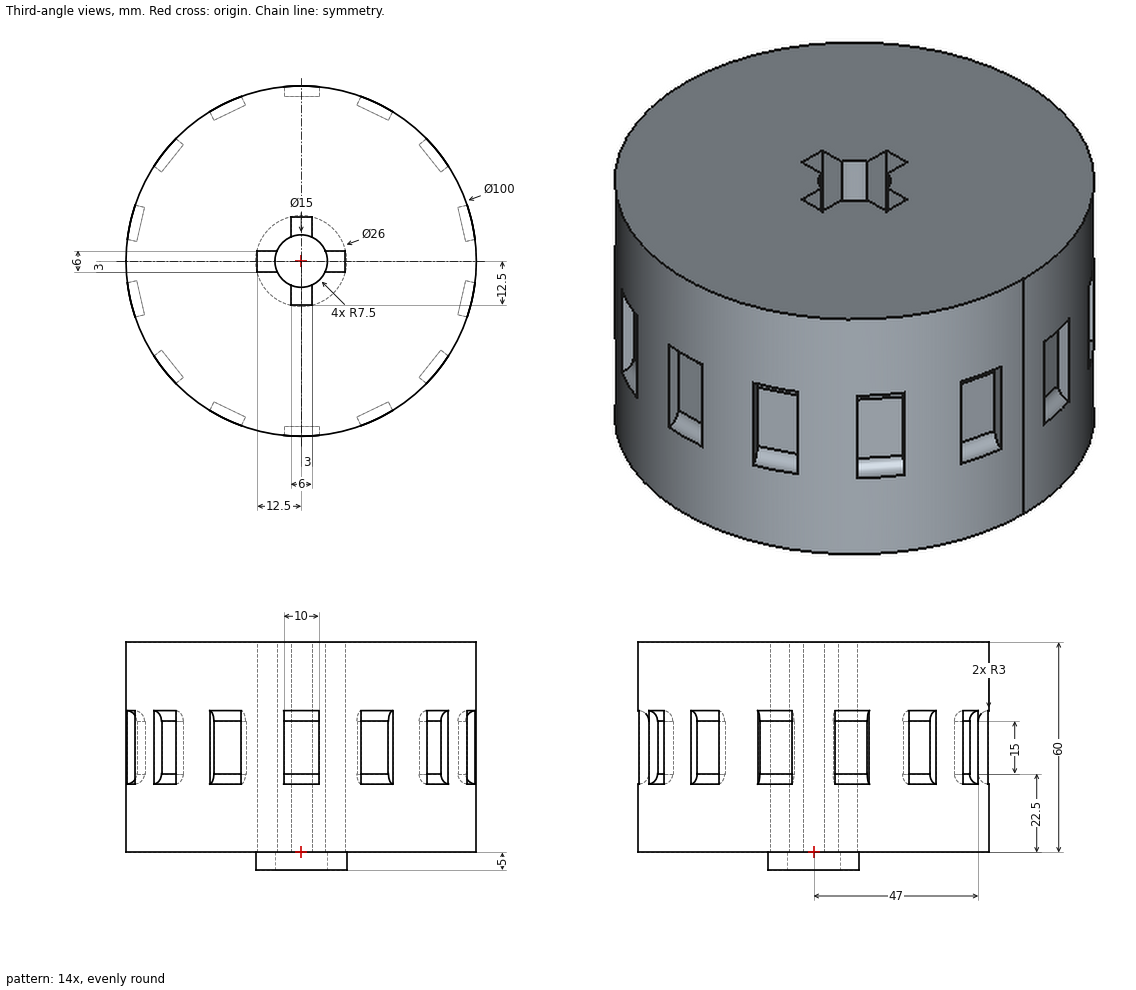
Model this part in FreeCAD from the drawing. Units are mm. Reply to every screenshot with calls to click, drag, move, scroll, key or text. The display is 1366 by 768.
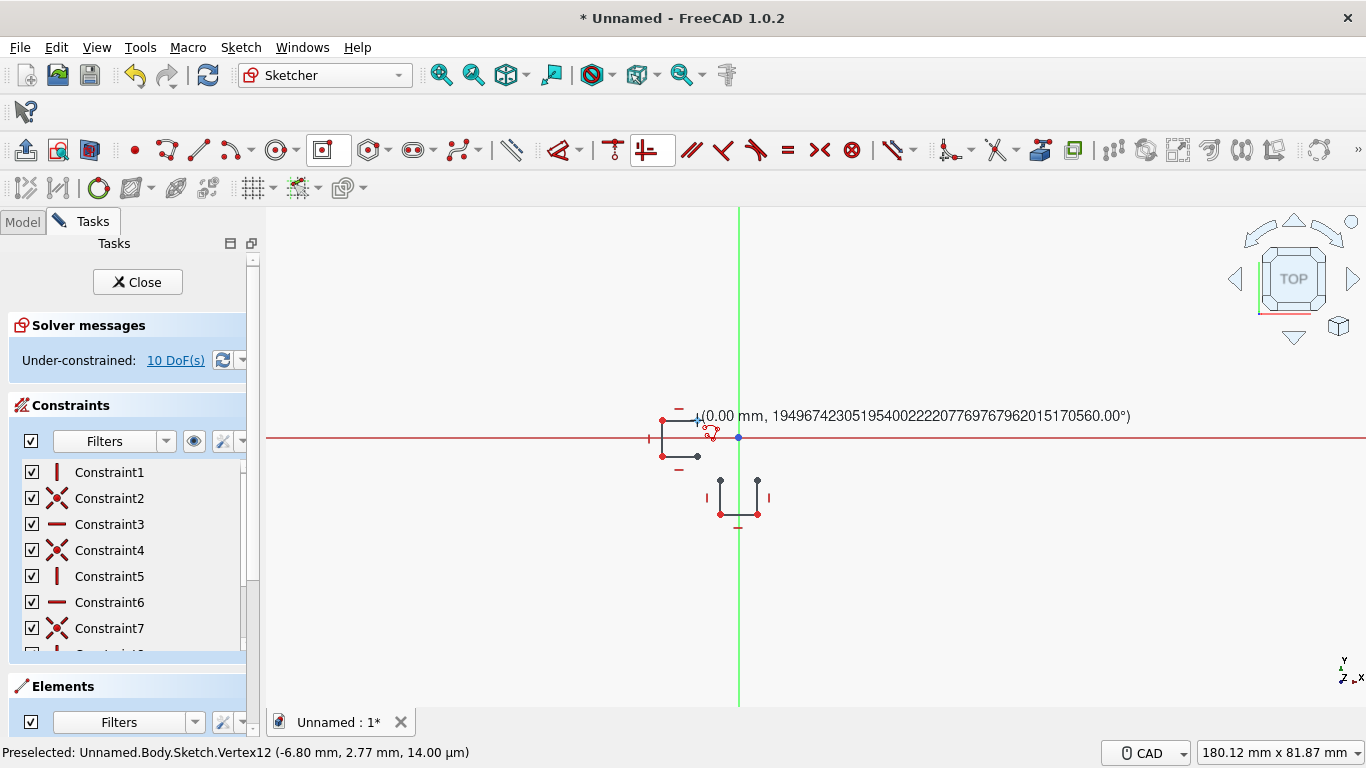
click(720, 396)
click(720, 362)
click(757, 362)
click(757, 396)
right_click(757, 396)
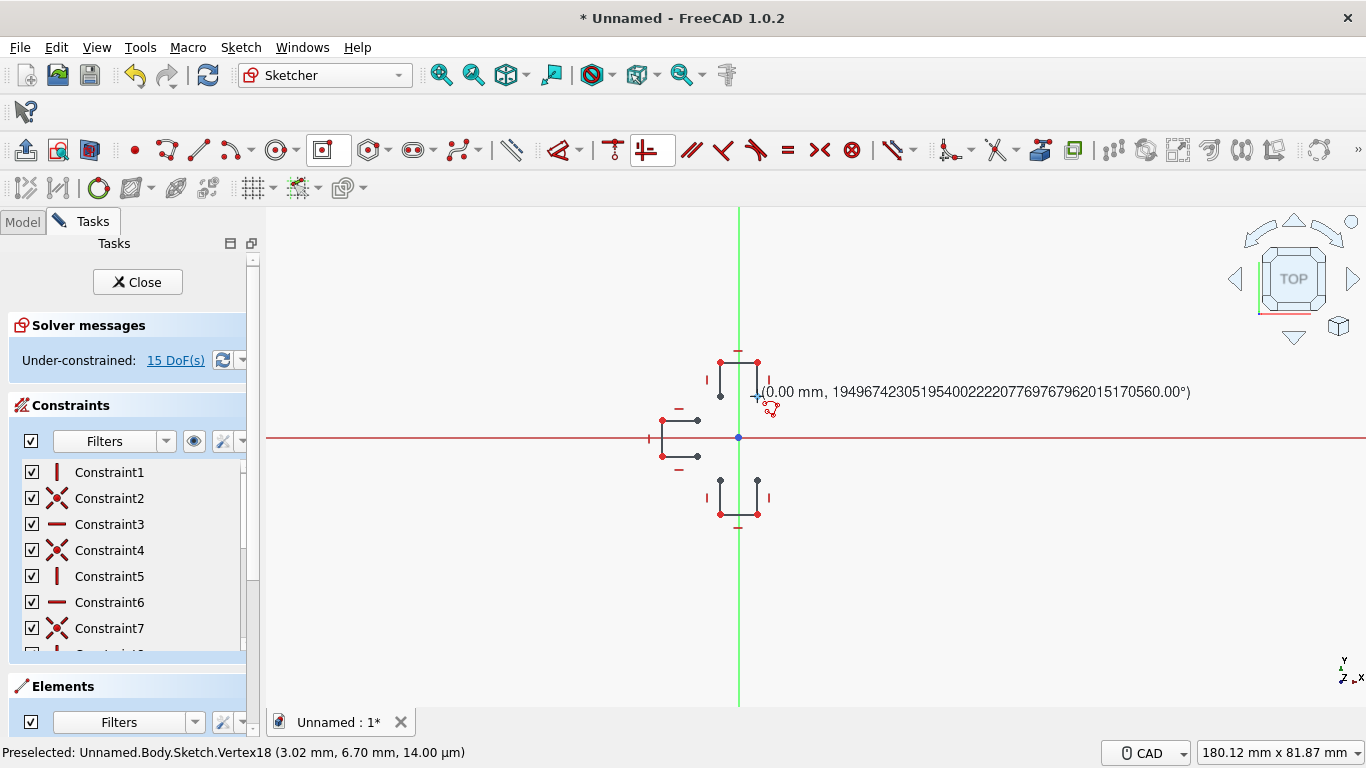
click(781, 420)
click(815, 420)
click(815, 456)
click(781, 456)
right_click(781, 456)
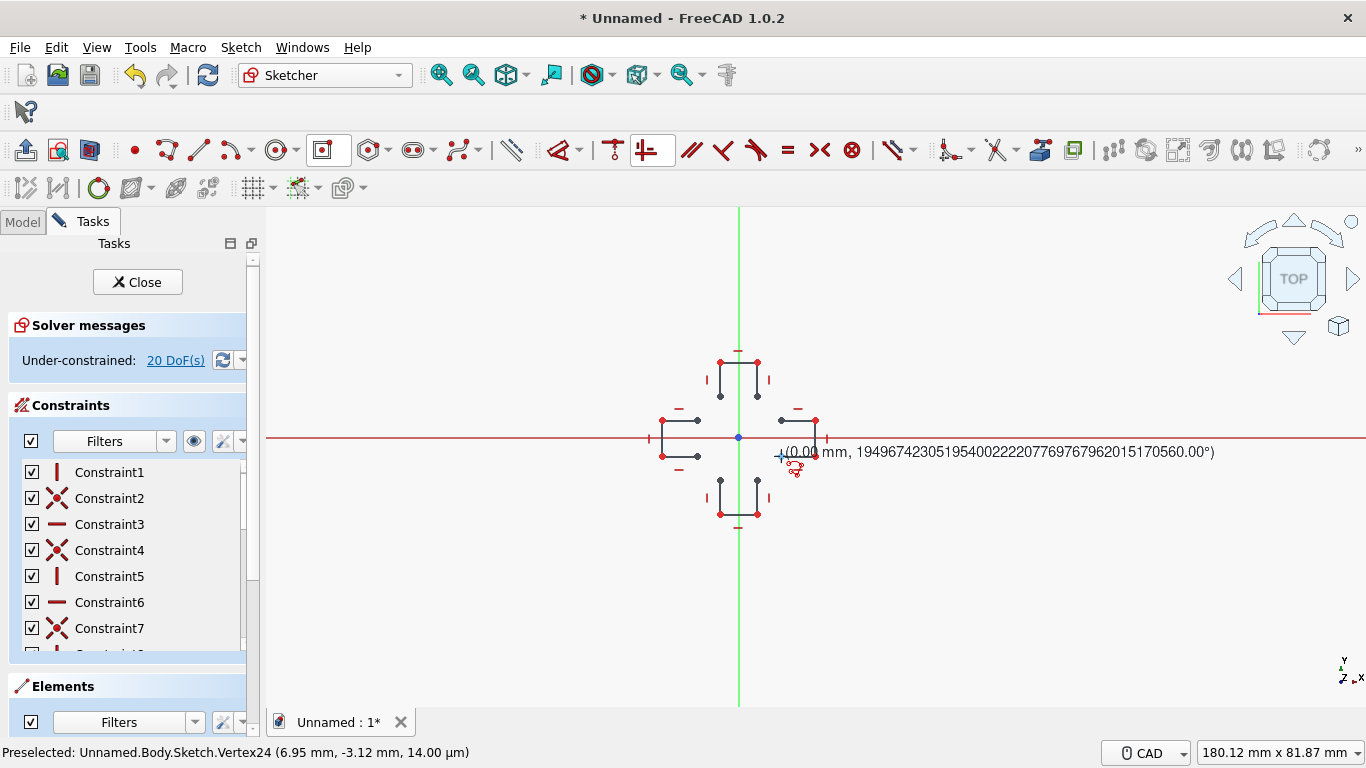
key(g)
key(3)
key(a)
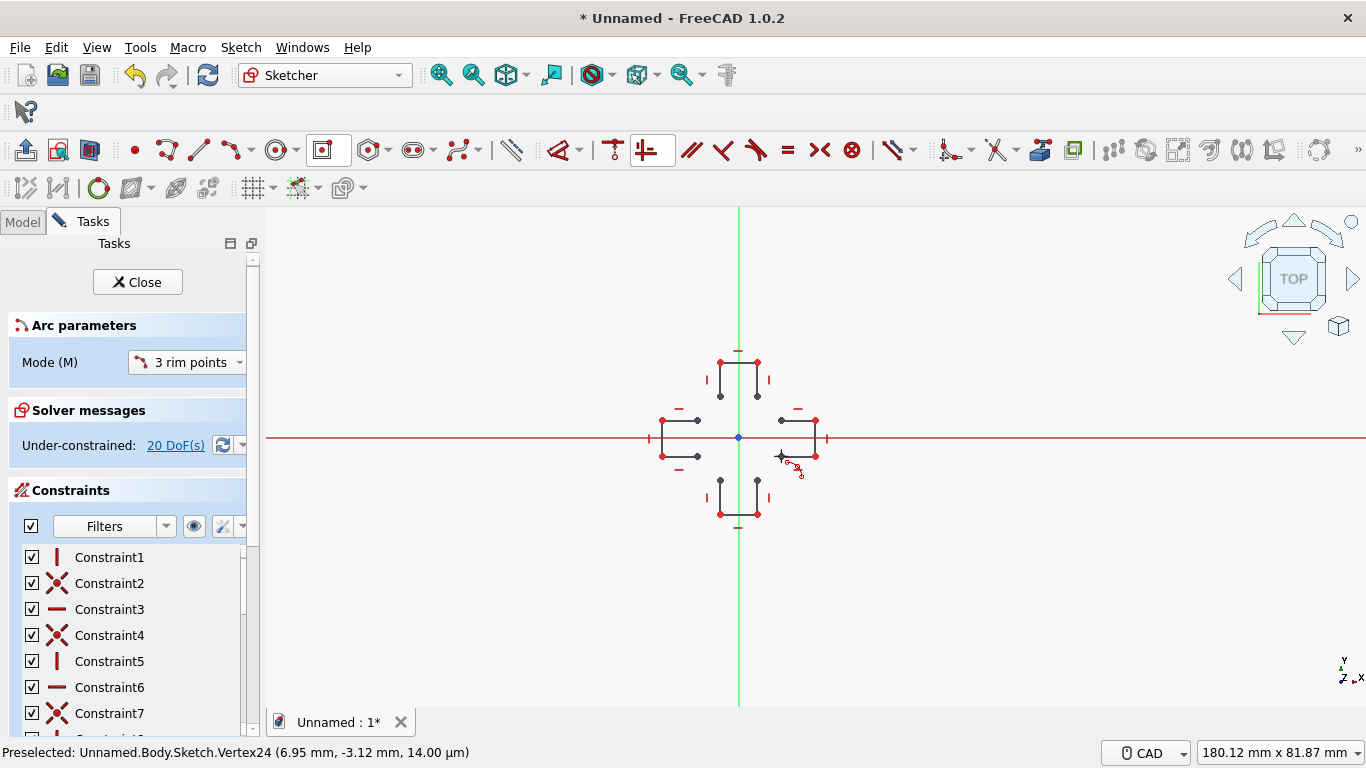
click(720, 481)
click(697, 457)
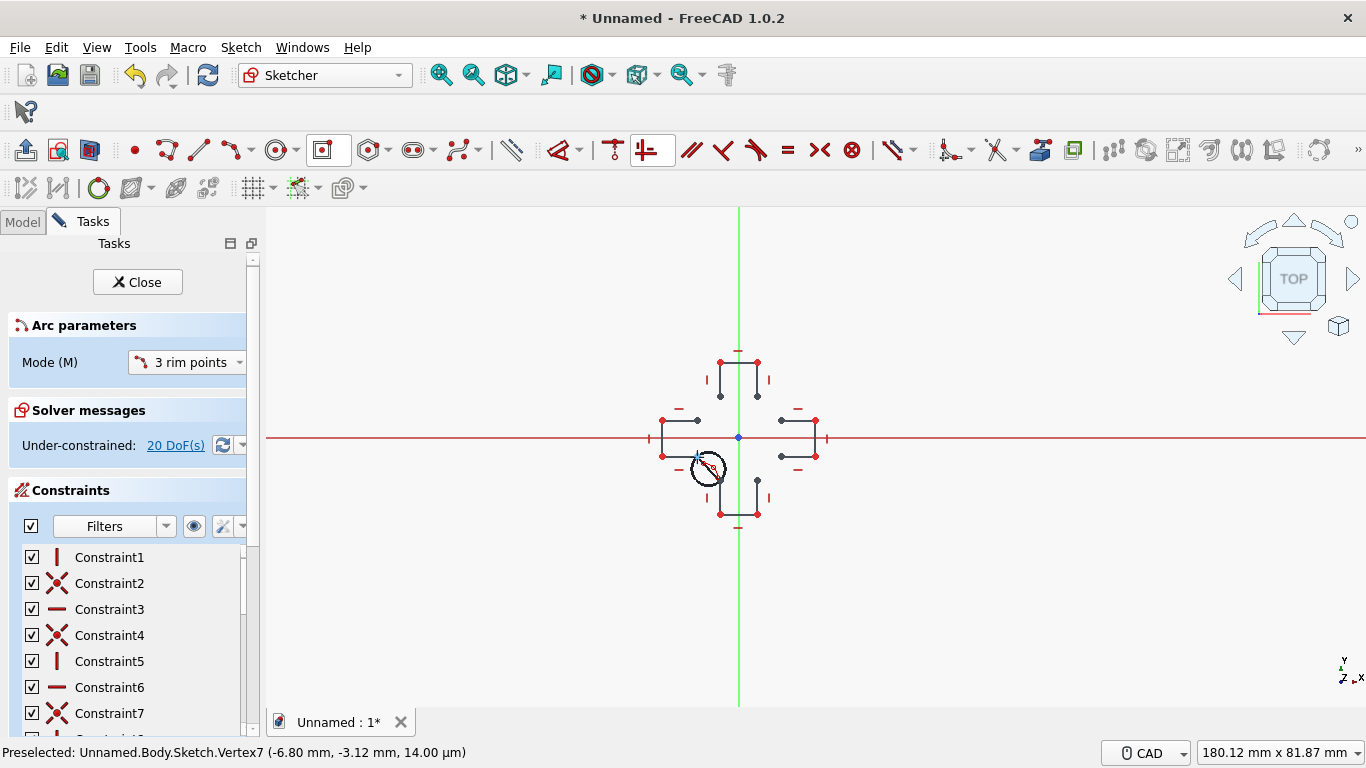
scroll(706, 470, up, 9)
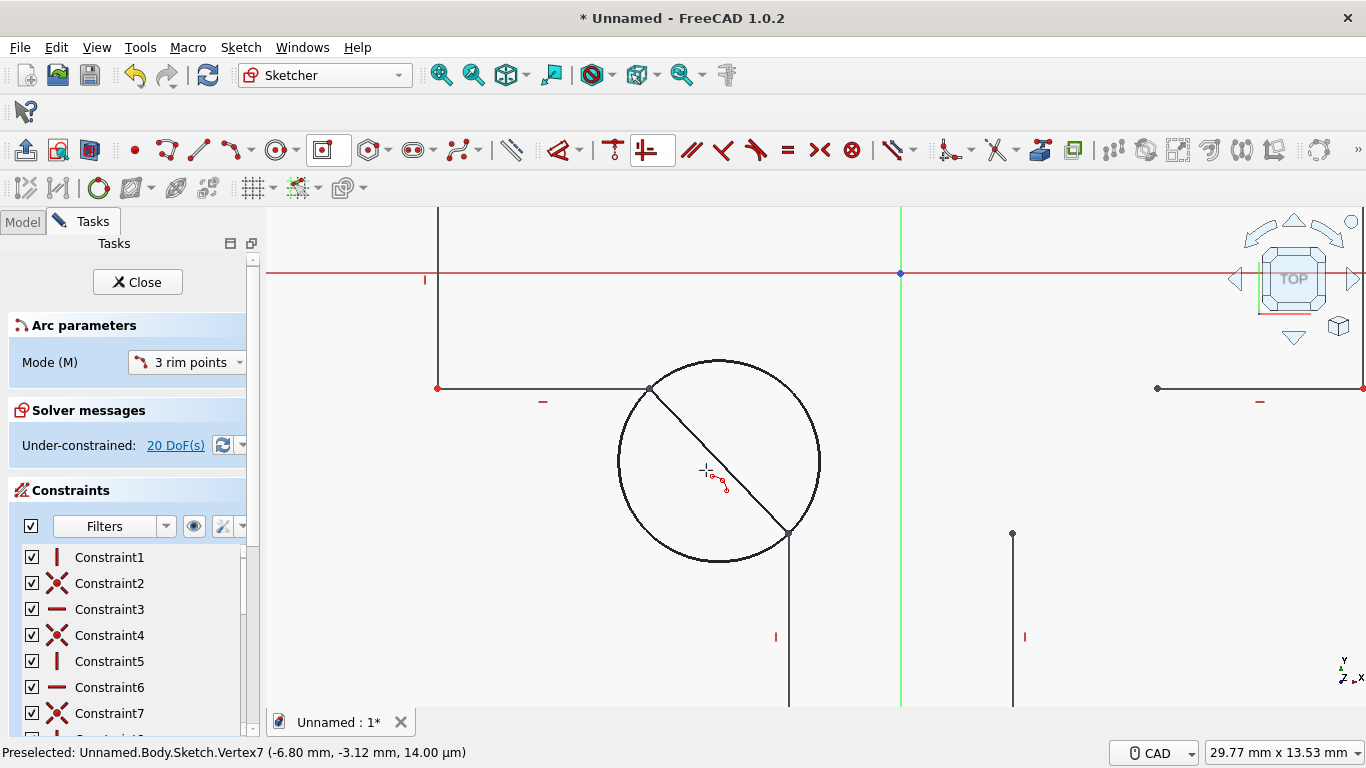
click(705, 469)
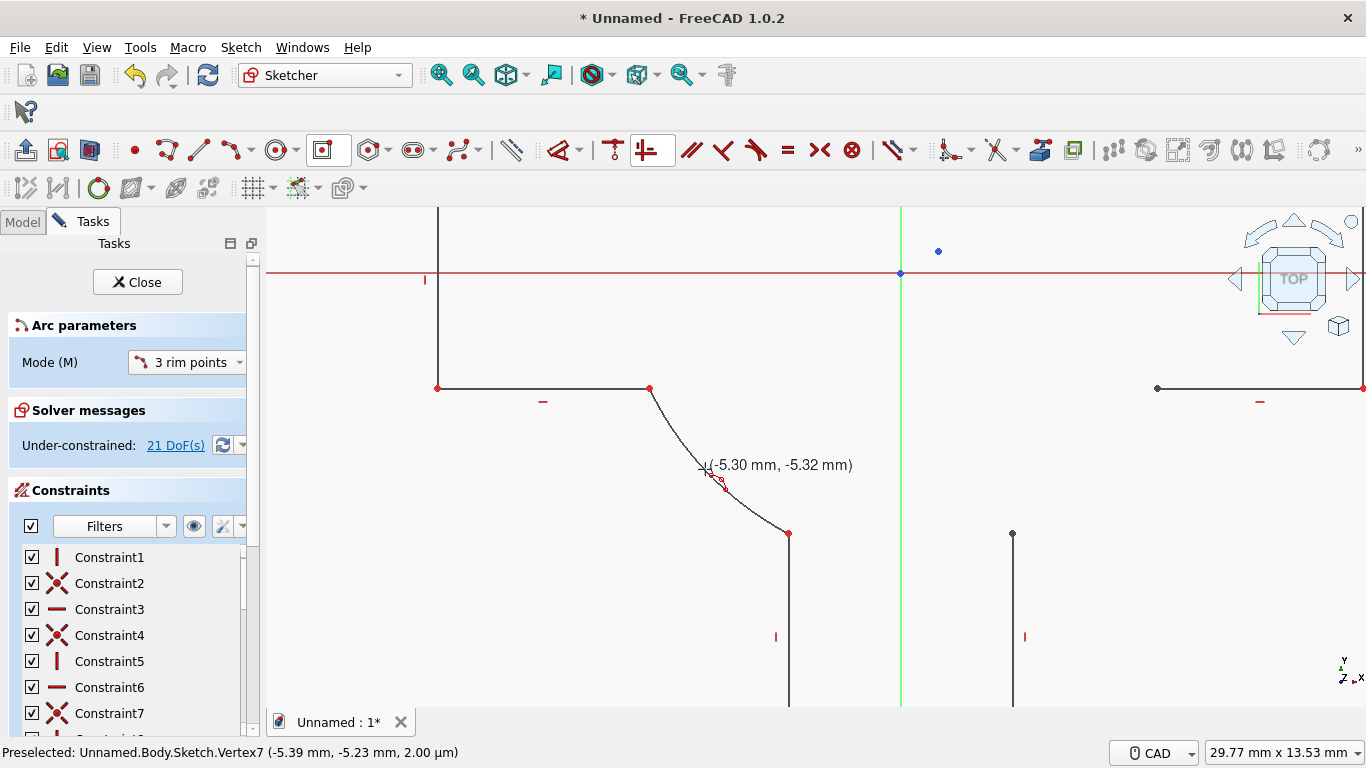
scroll(732, 475, down, 12)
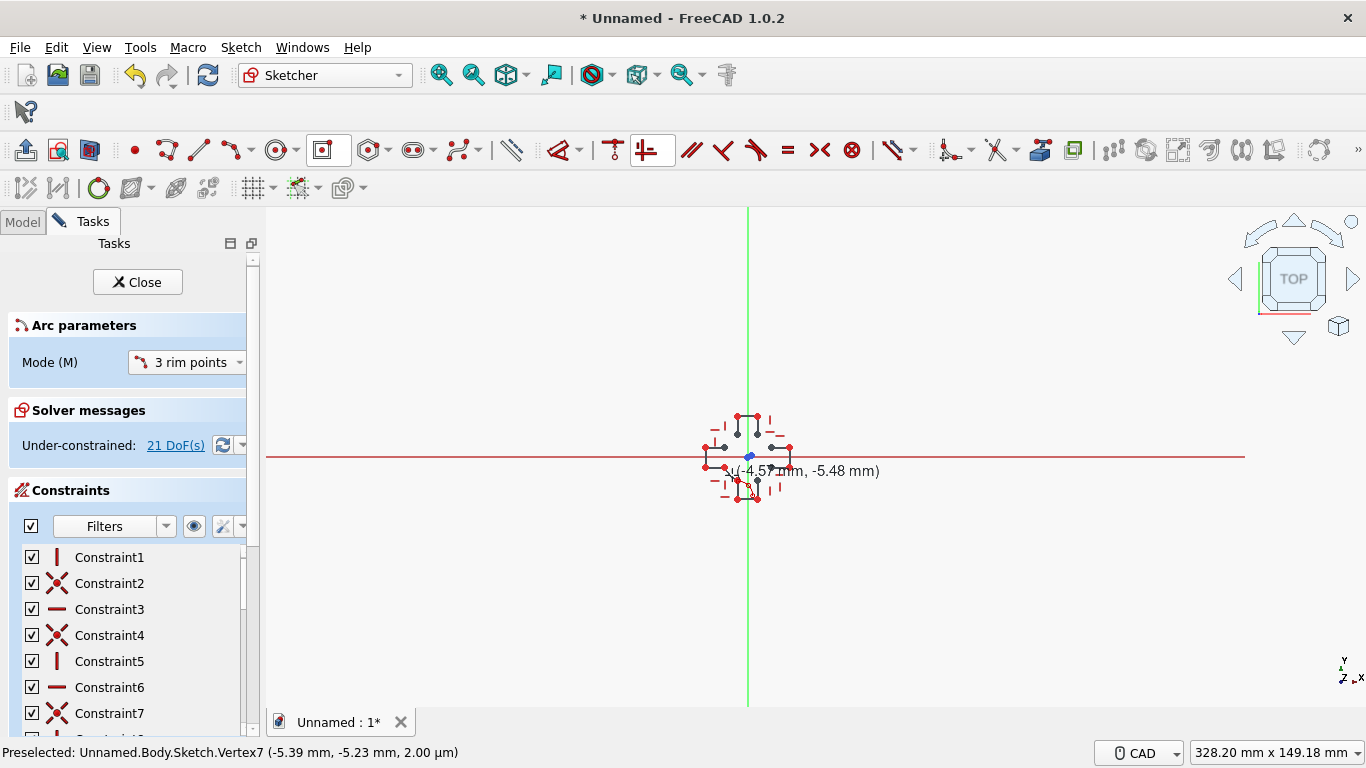
scroll(725, 447, up, 3)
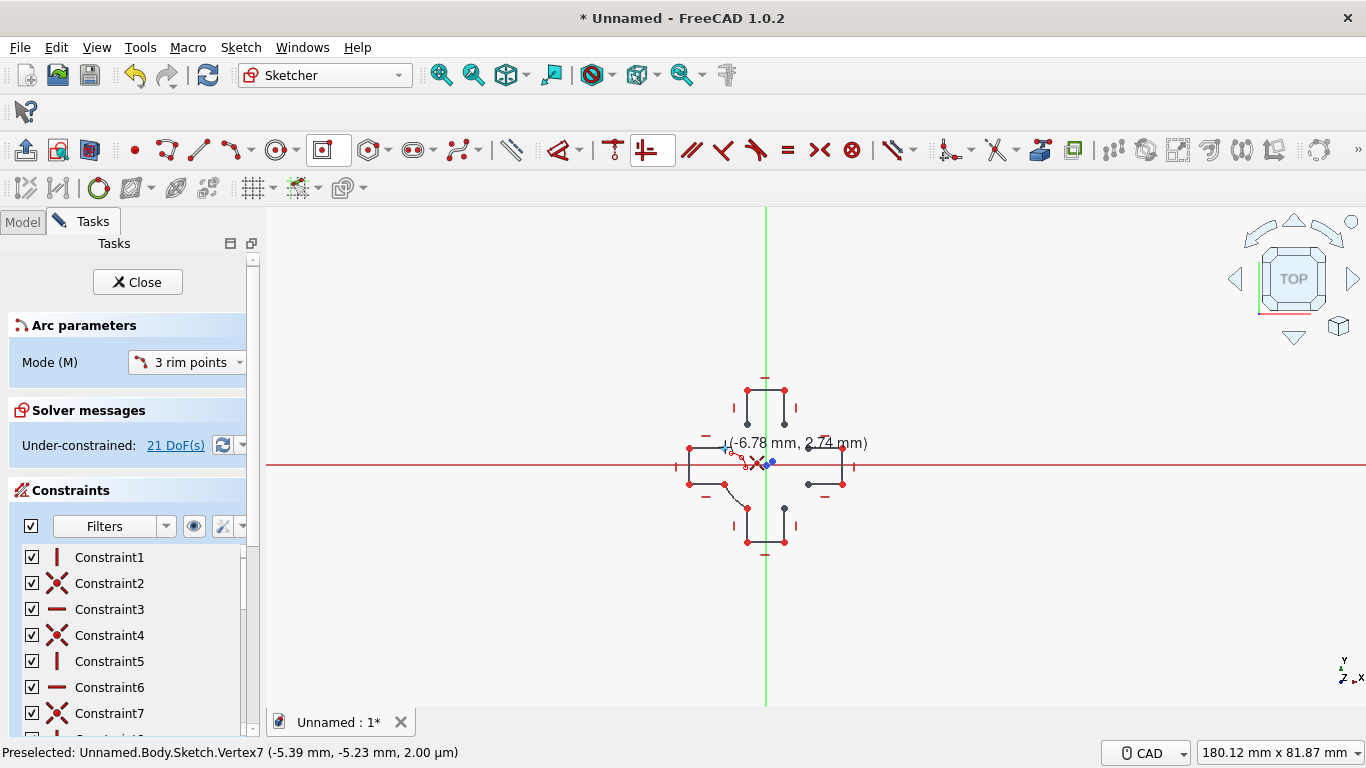
click(724, 448)
click(747, 424)